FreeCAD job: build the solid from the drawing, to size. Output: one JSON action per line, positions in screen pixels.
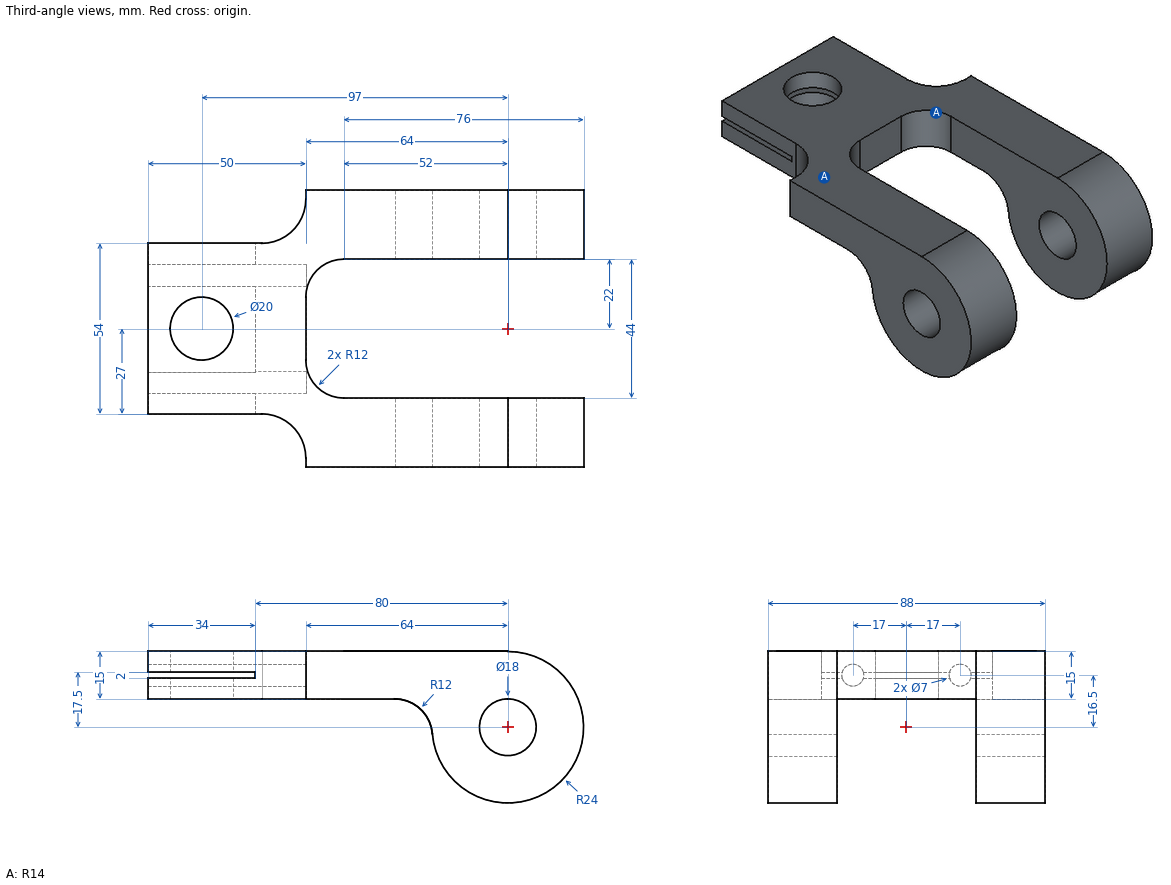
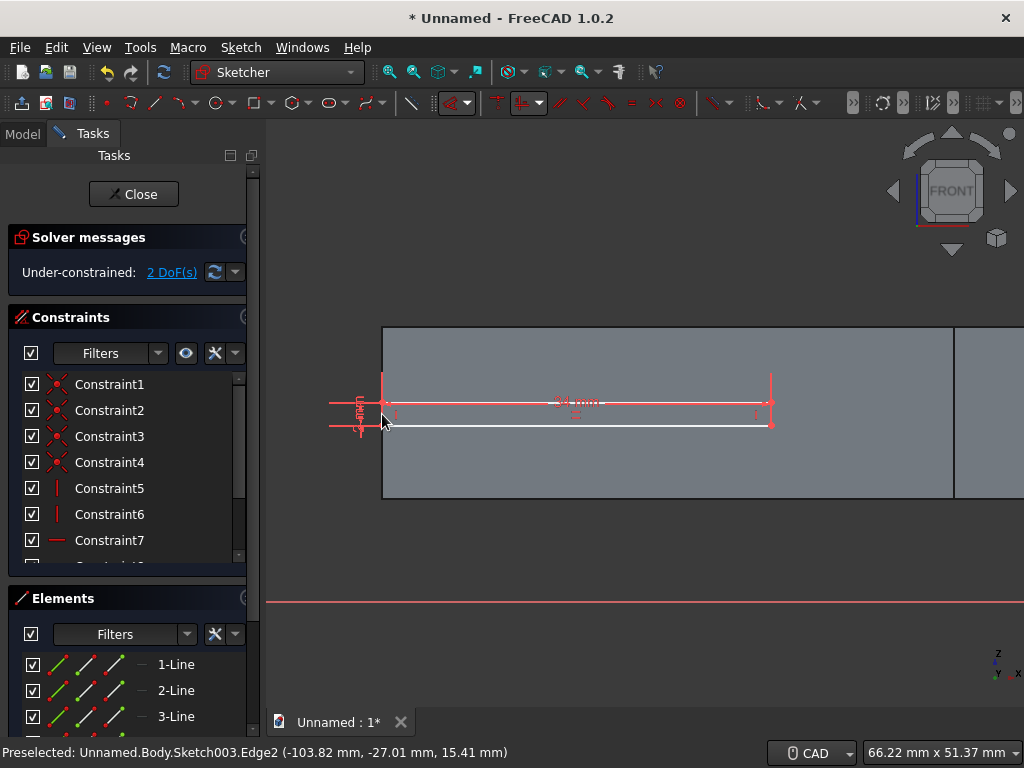
{"action": "left_click", "coordinate": [771, 426]}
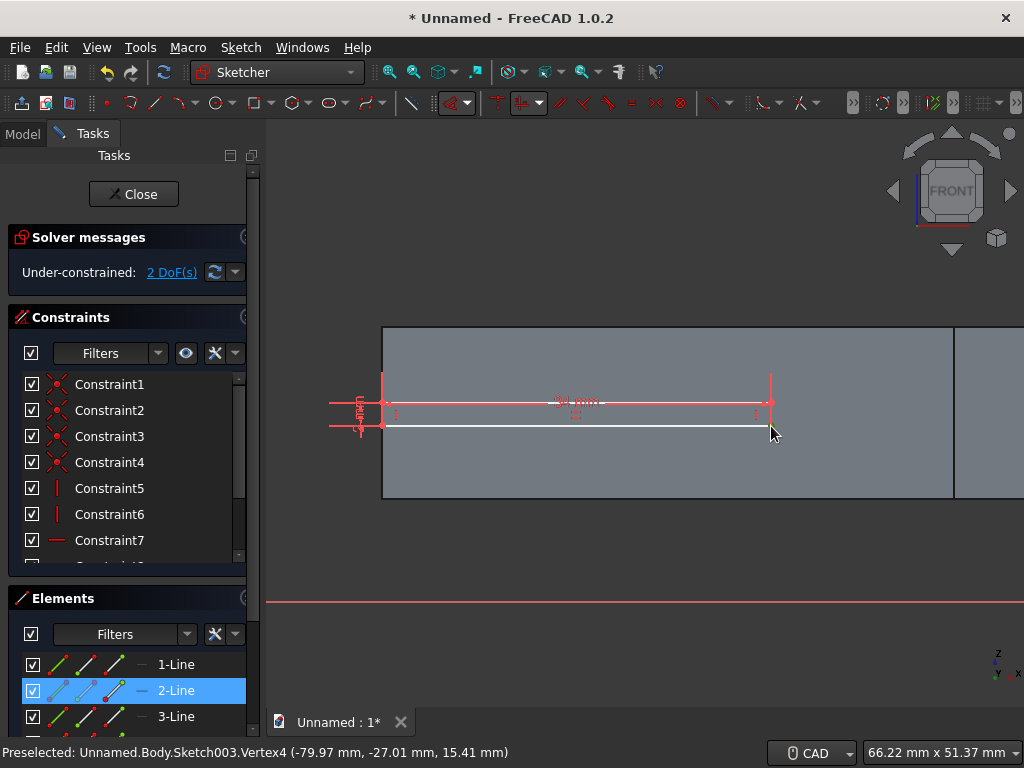
{"action": "left_click", "coordinate": [470, 104]}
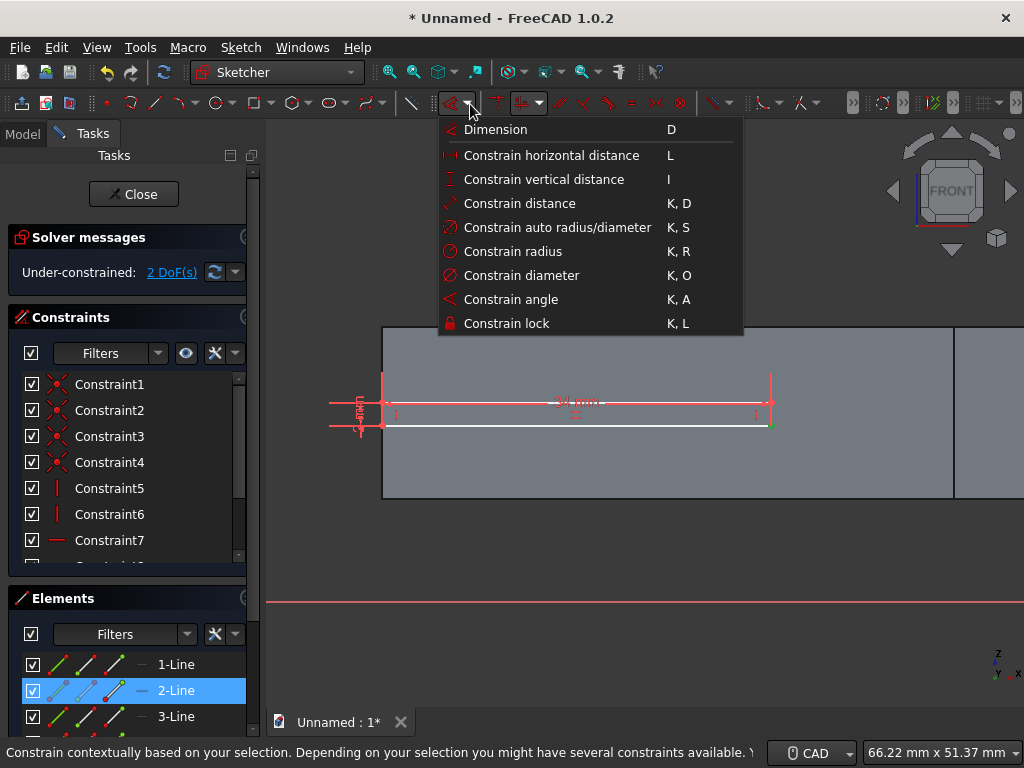
{"action": "left_click", "coordinate": [591, 155]}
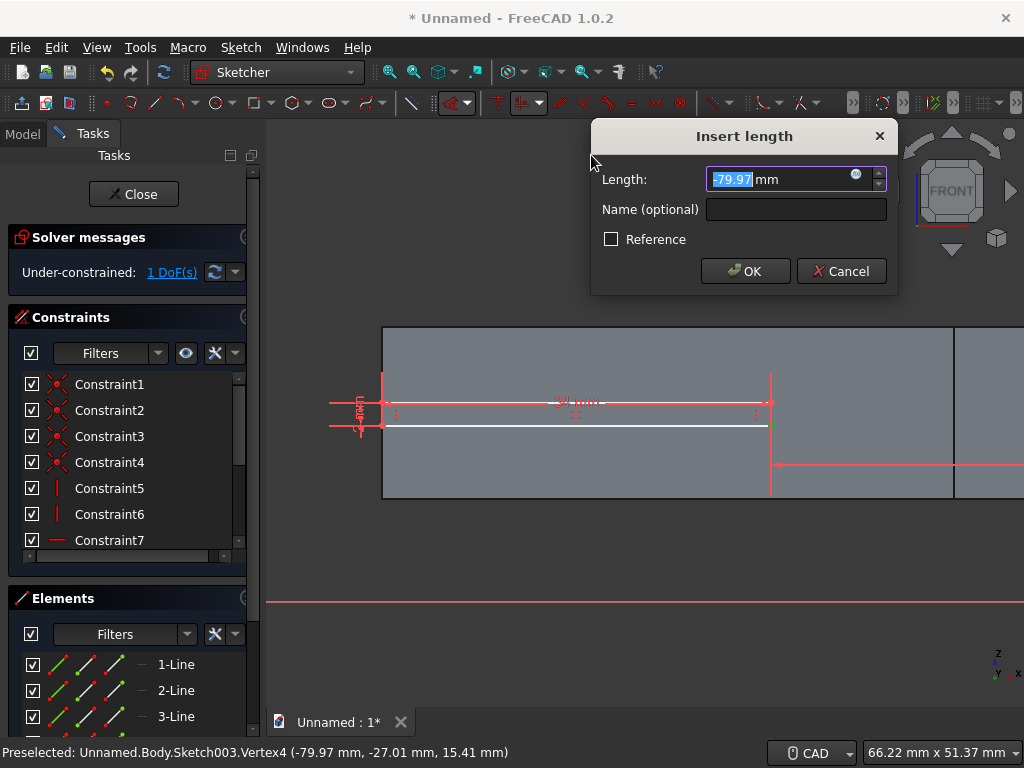
{"action": "type", "text": "-80"}
{"action": "key", "text": "Return"}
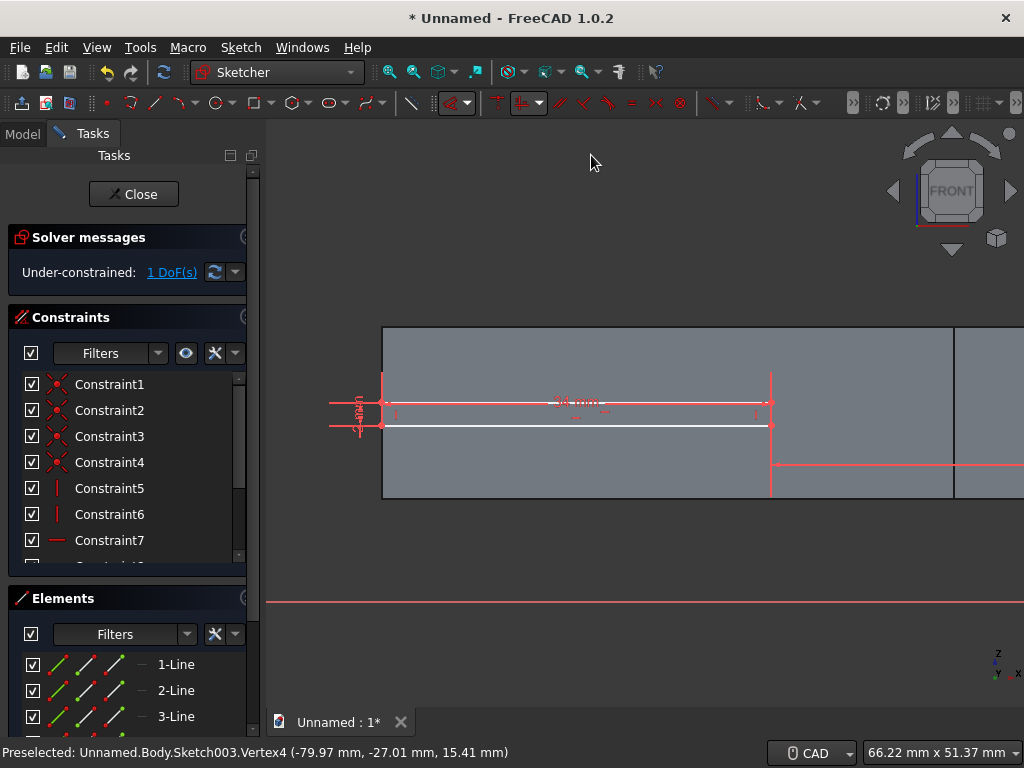
{"action": "left_click", "coordinate": [382, 403]}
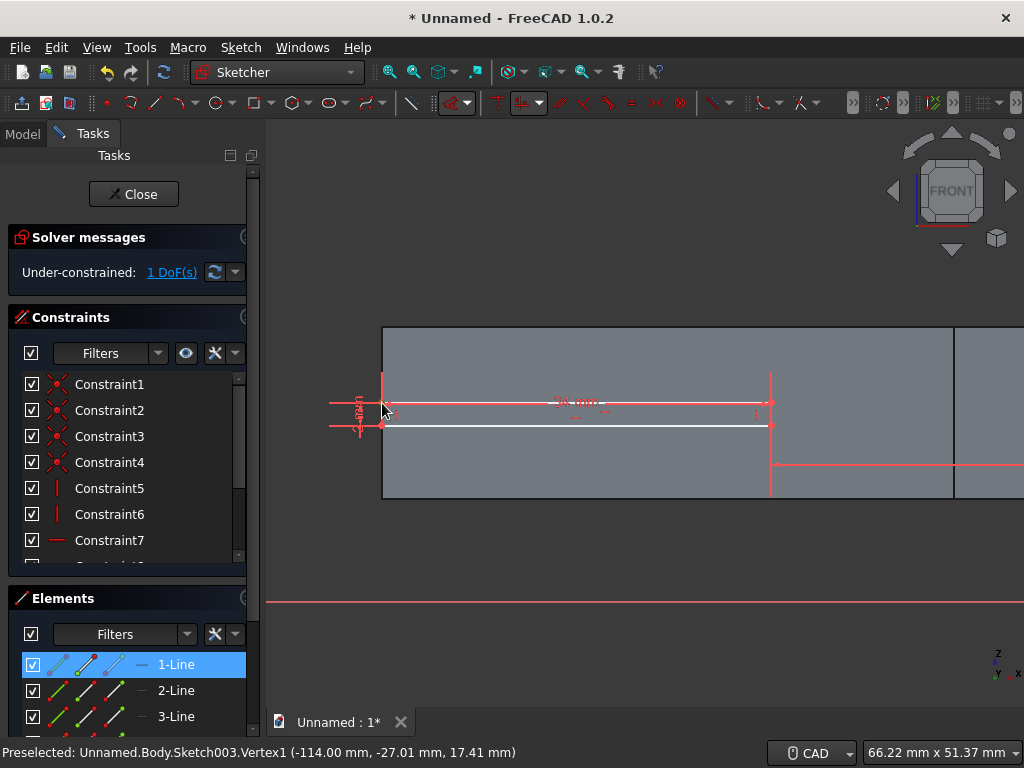
{"action": "key", "text": "i"}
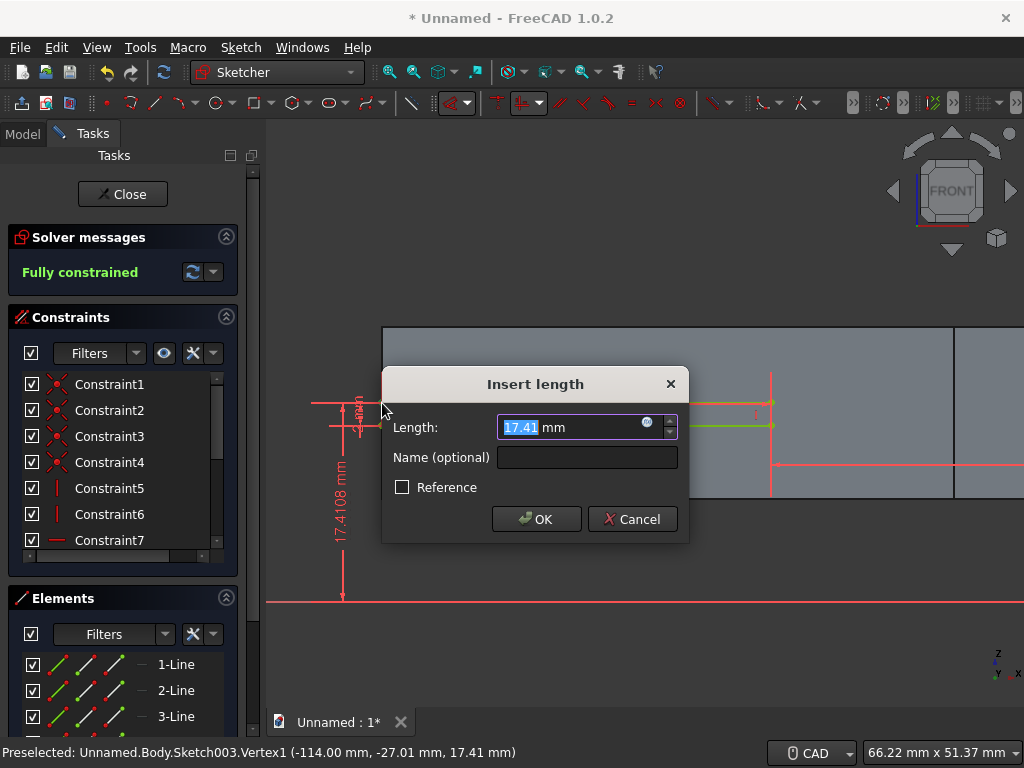
{"action": "type", "text": "17.5"}
{"action": "key", "text": "Return"}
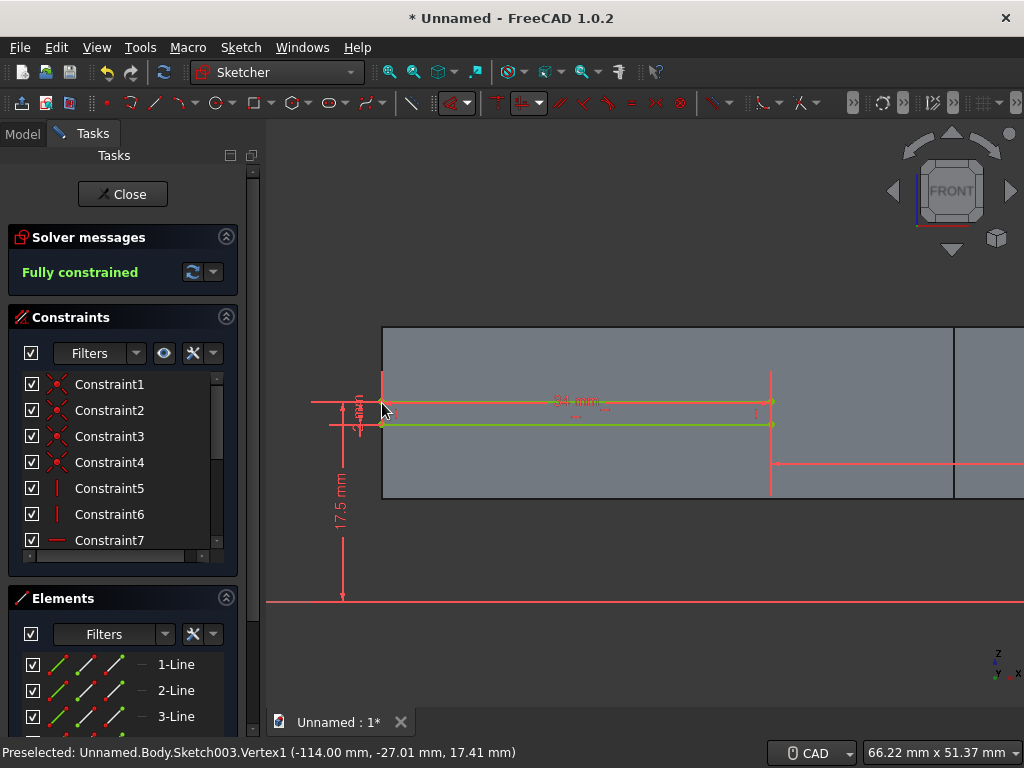
{"action": "left_click", "coordinate": [123, 194]}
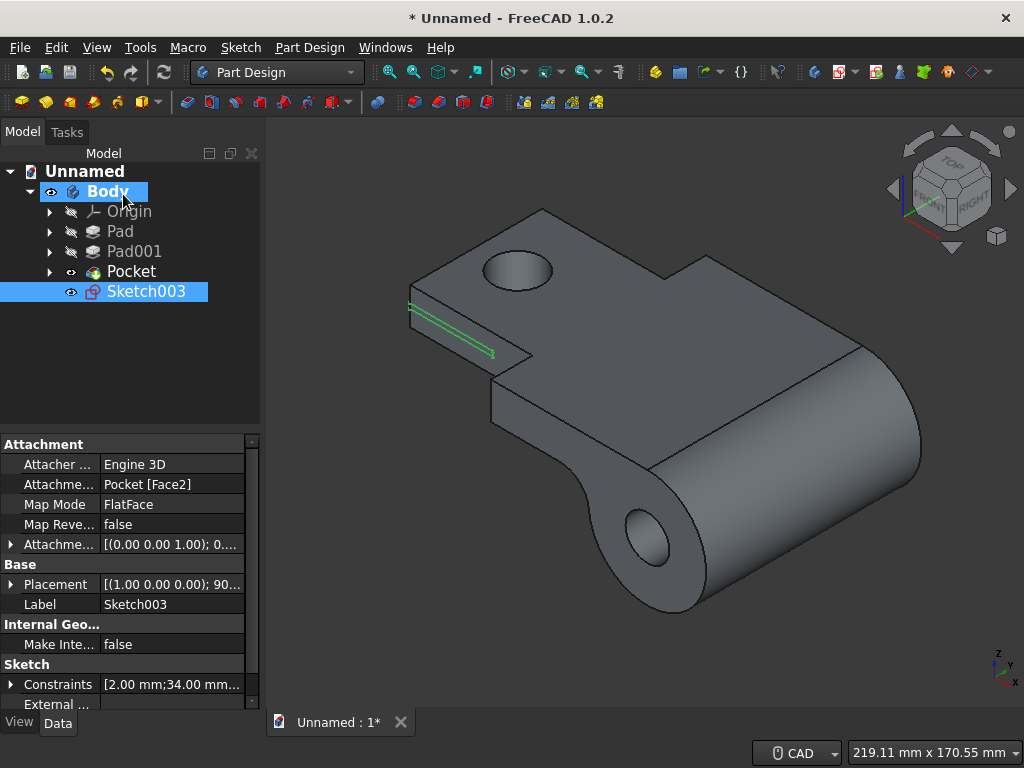
{"action": "left_click", "coordinate": [188, 102]}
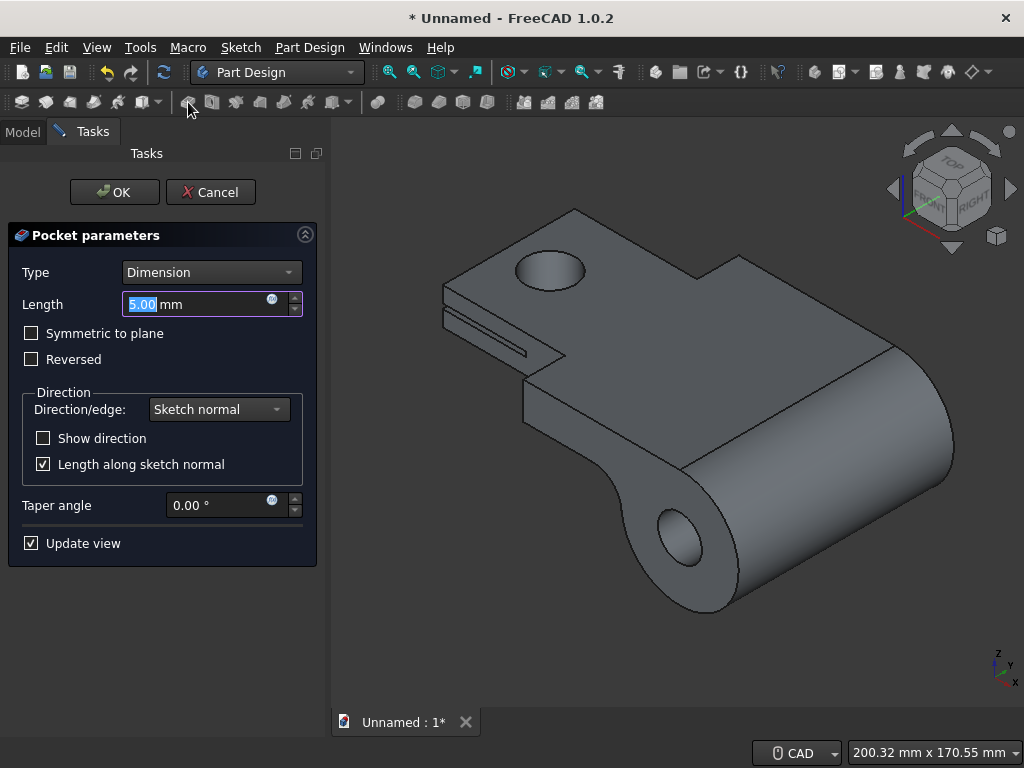
{"action": "left_click", "coordinate": [212, 272]}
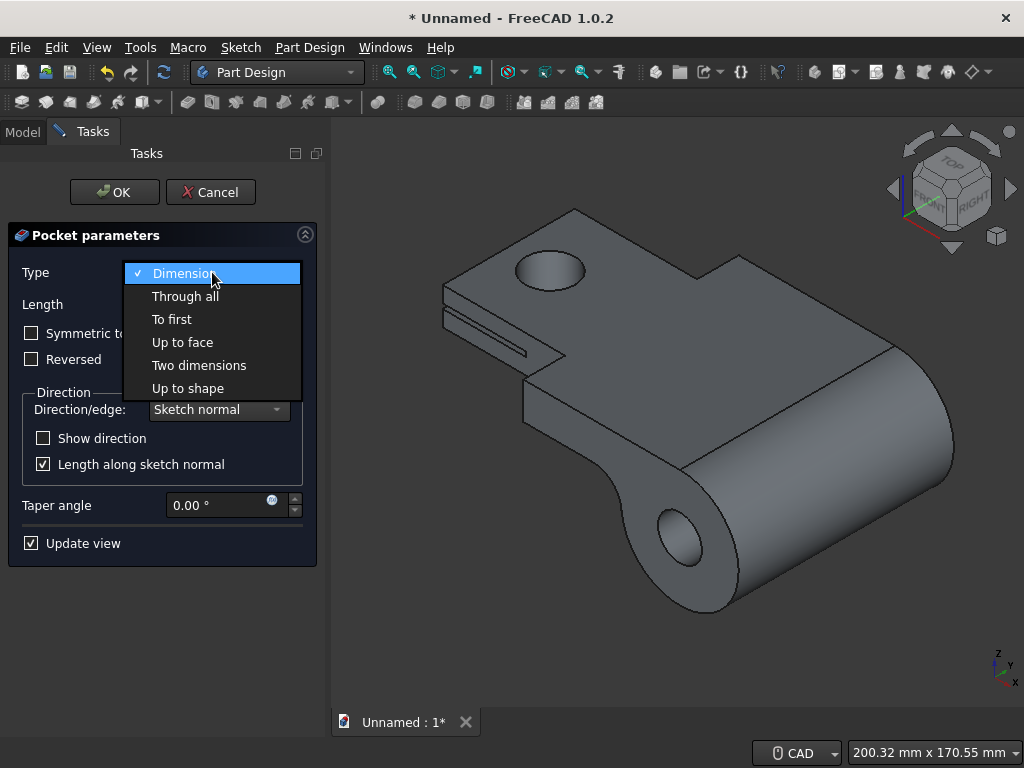
{"action": "left_click", "coordinate": [212, 320]}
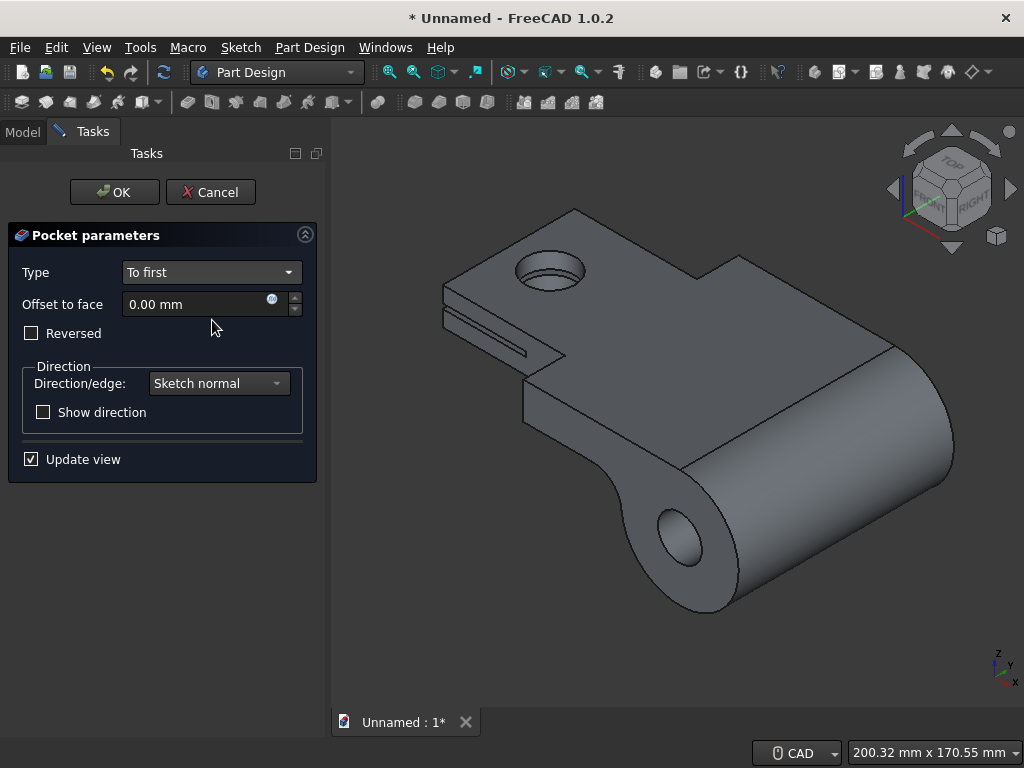
{"action": "left_click", "coordinate": [115, 192]}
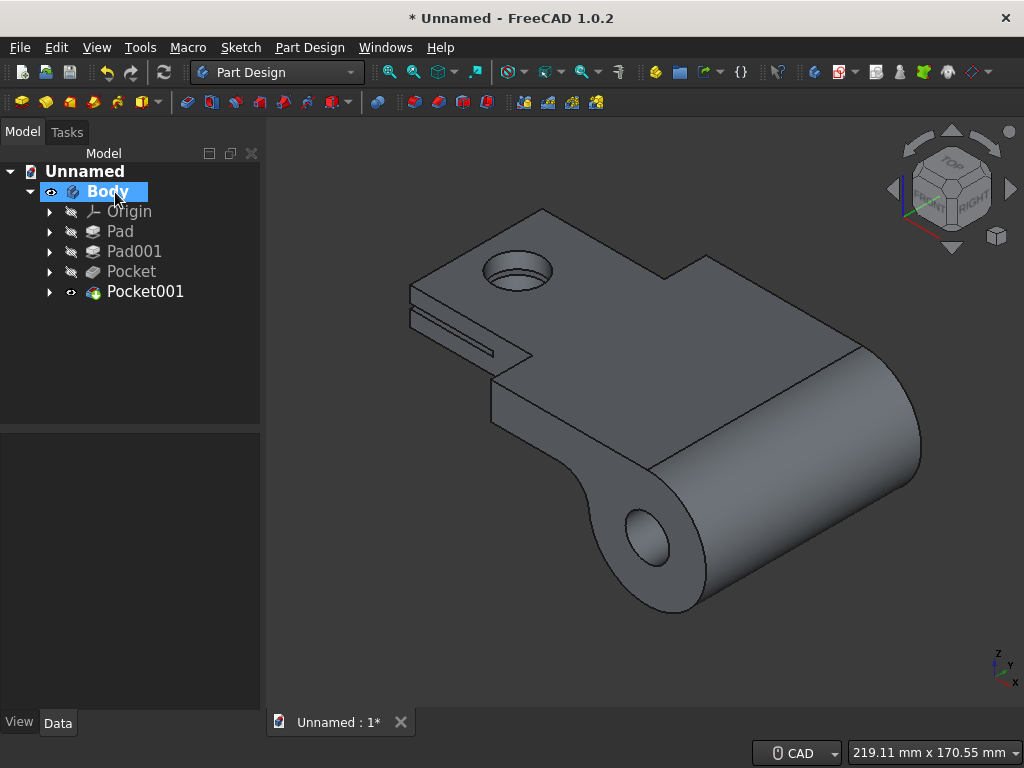
{"action": "key", "text": "2"}